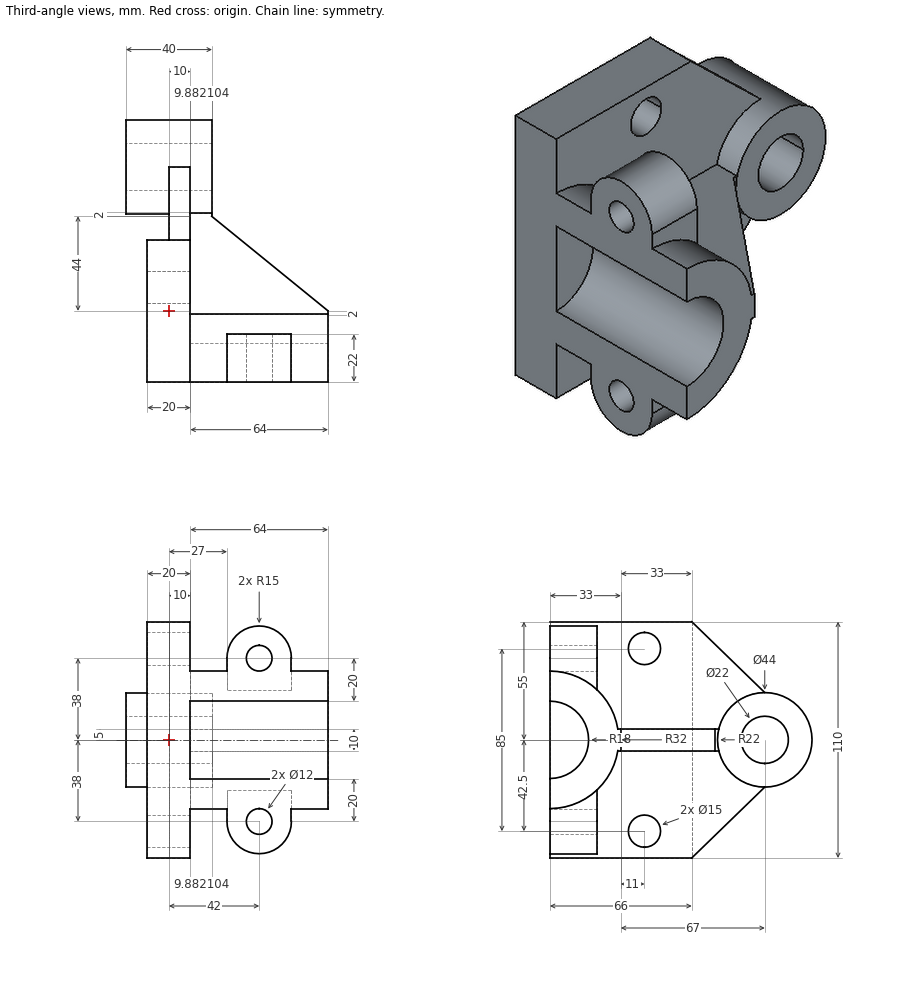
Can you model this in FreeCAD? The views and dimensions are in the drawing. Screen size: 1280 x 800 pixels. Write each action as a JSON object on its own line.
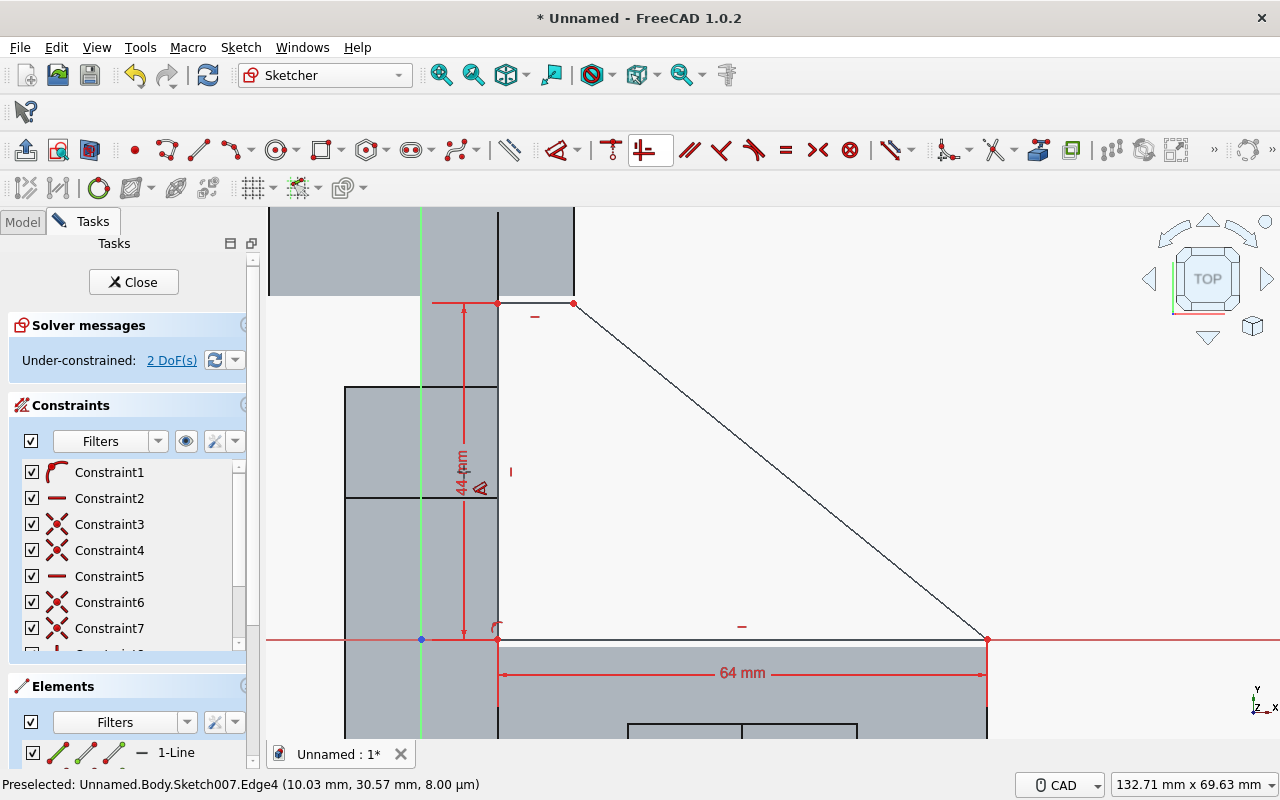
{"action": "left_click", "coordinate": [498, 640]}
{"action": "left_click", "coordinate": [460, 674]}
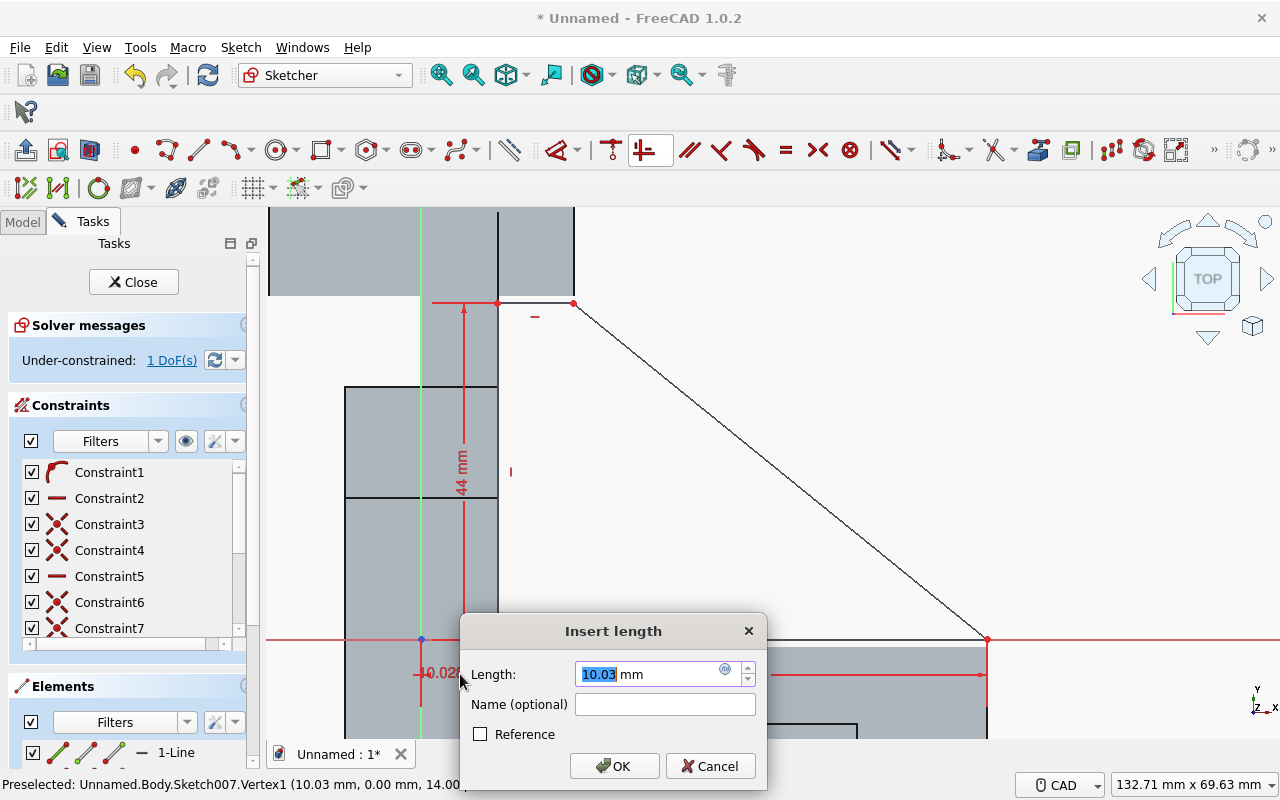
{"action": "type", "text": "10"}
{"action": "key", "text": "Return"}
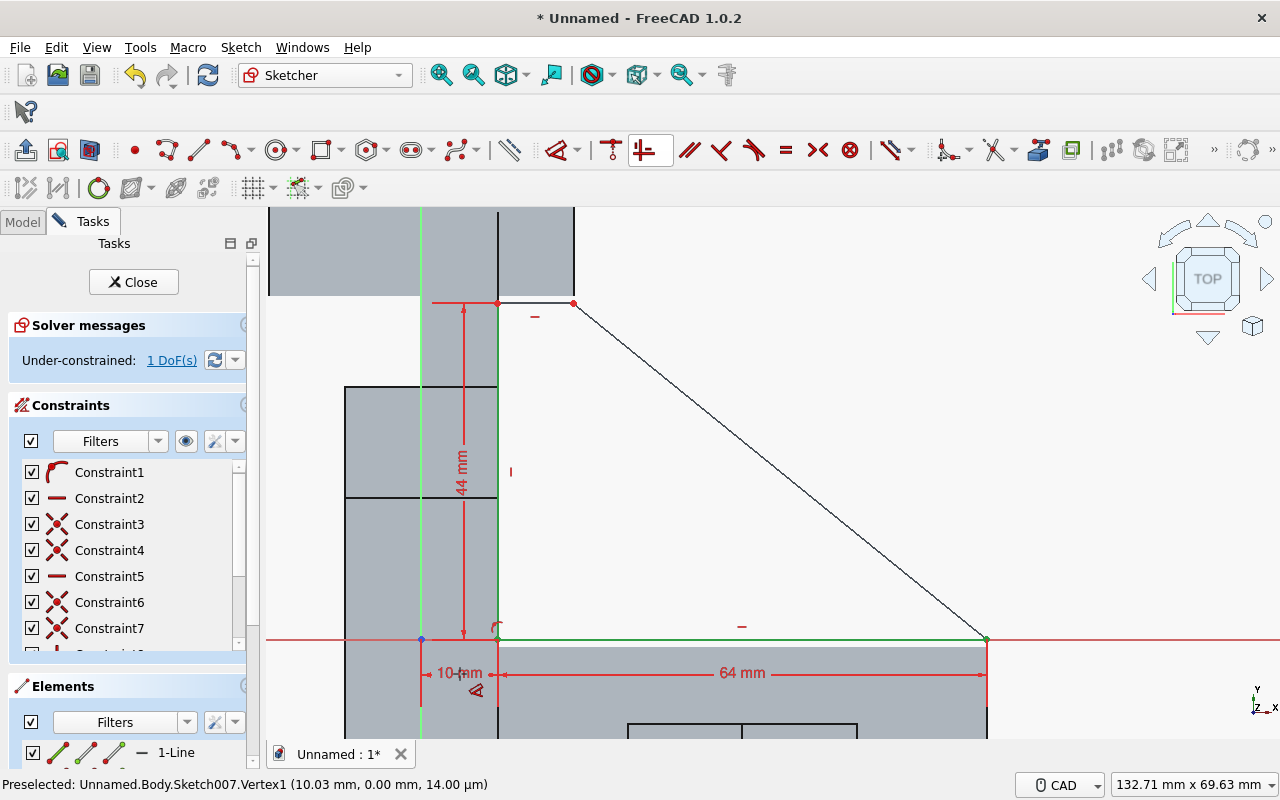
{"action": "left_click", "coordinate": [550, 303]}
{"action": "left_click", "coordinate": [535, 269]}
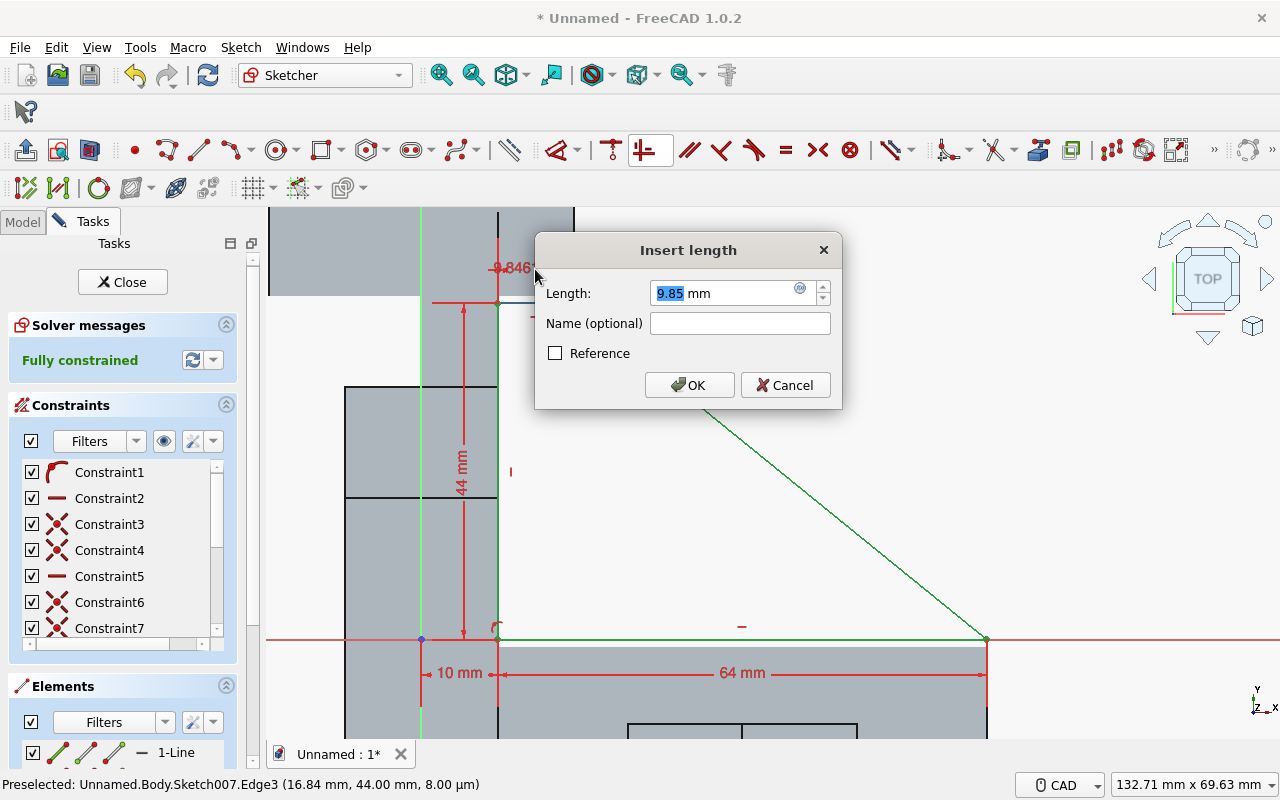
{"action": "type", "text": "9.882104"}
{"action": "key", "text": "Return"}
{"action": "key", "text": "Escape"}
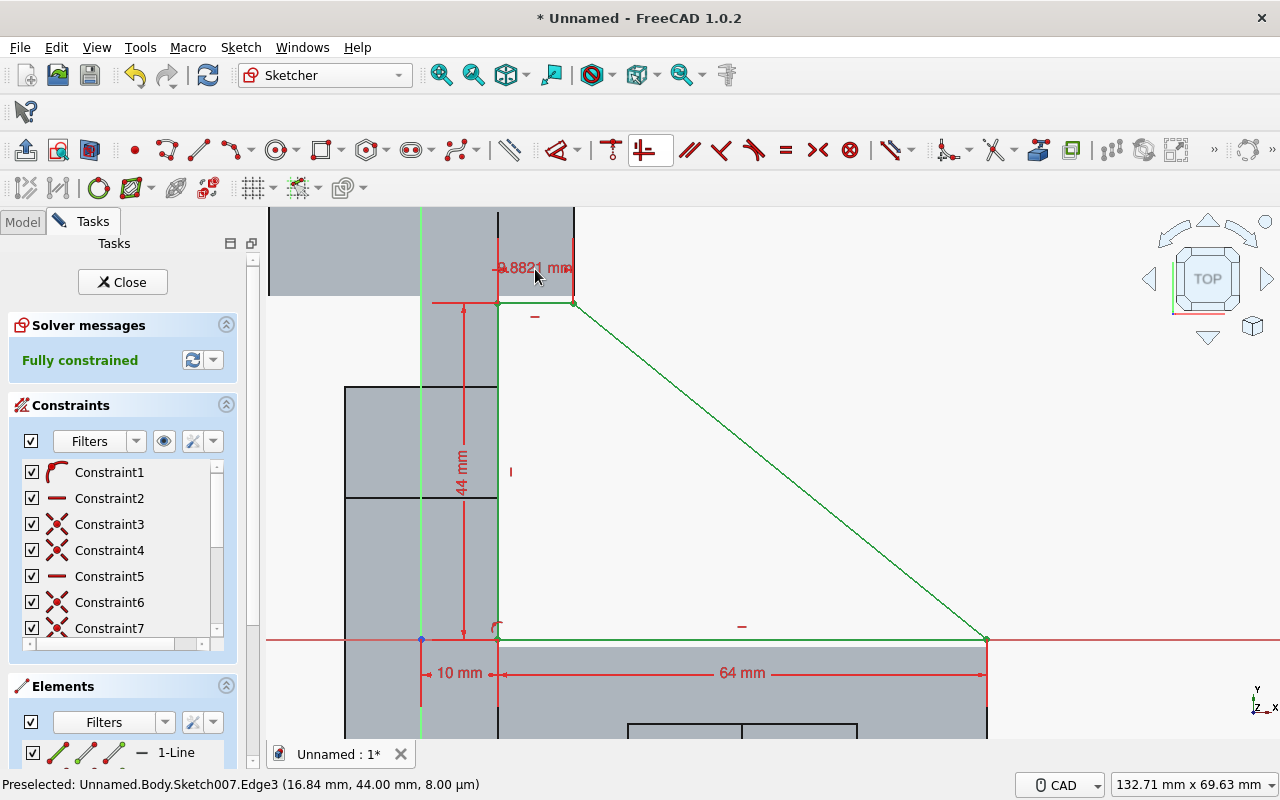
{"action": "left_click", "coordinate": [123, 282]}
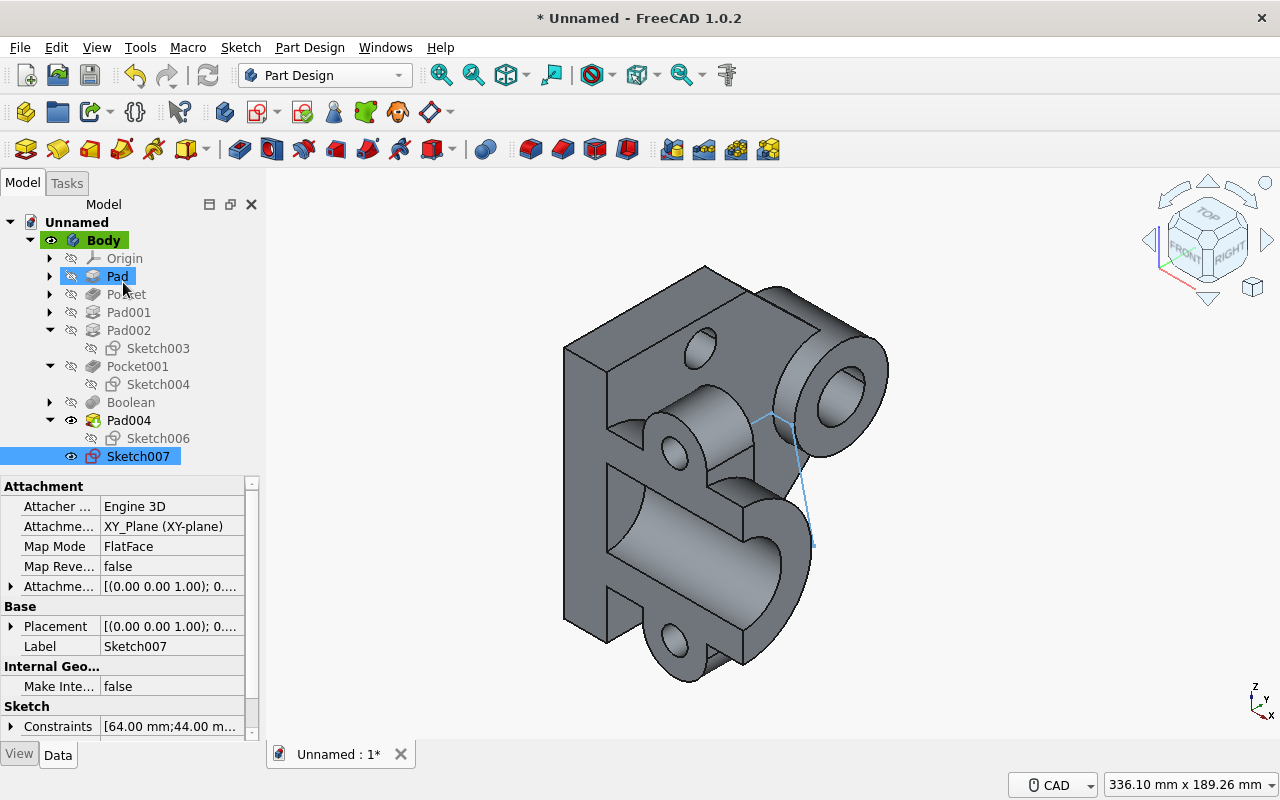
{"action": "left_click", "coordinate": [26, 150]}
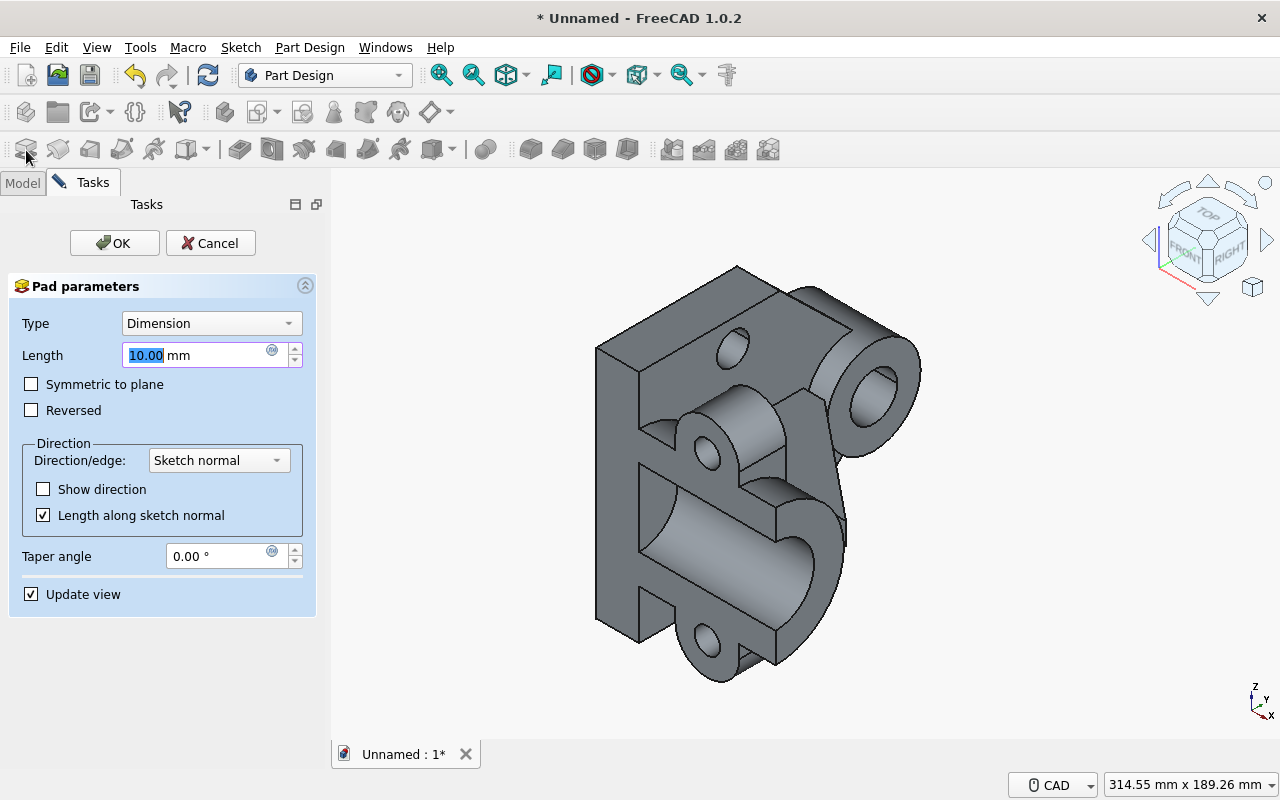
{"action": "type", "text": "10"}
{"action": "key", "text": "Tab"}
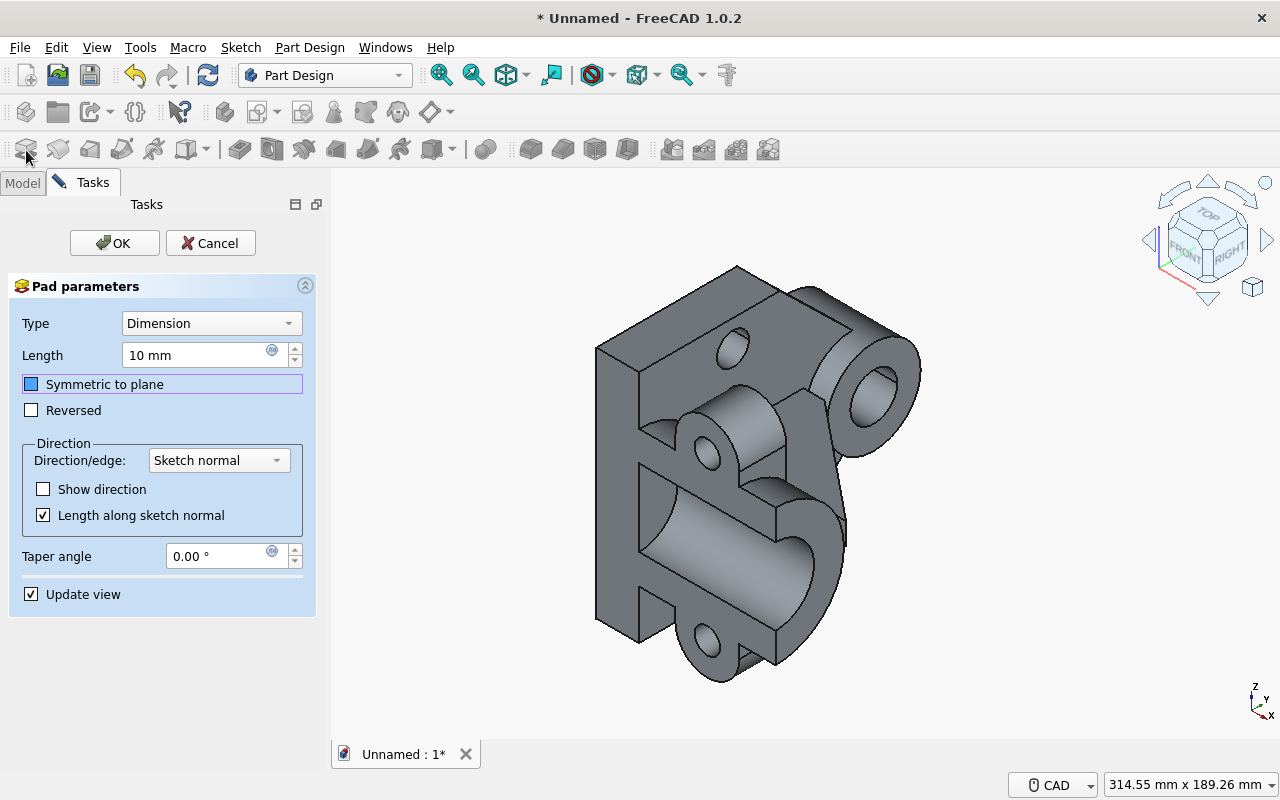
{"action": "left_click", "coordinate": [30, 384]}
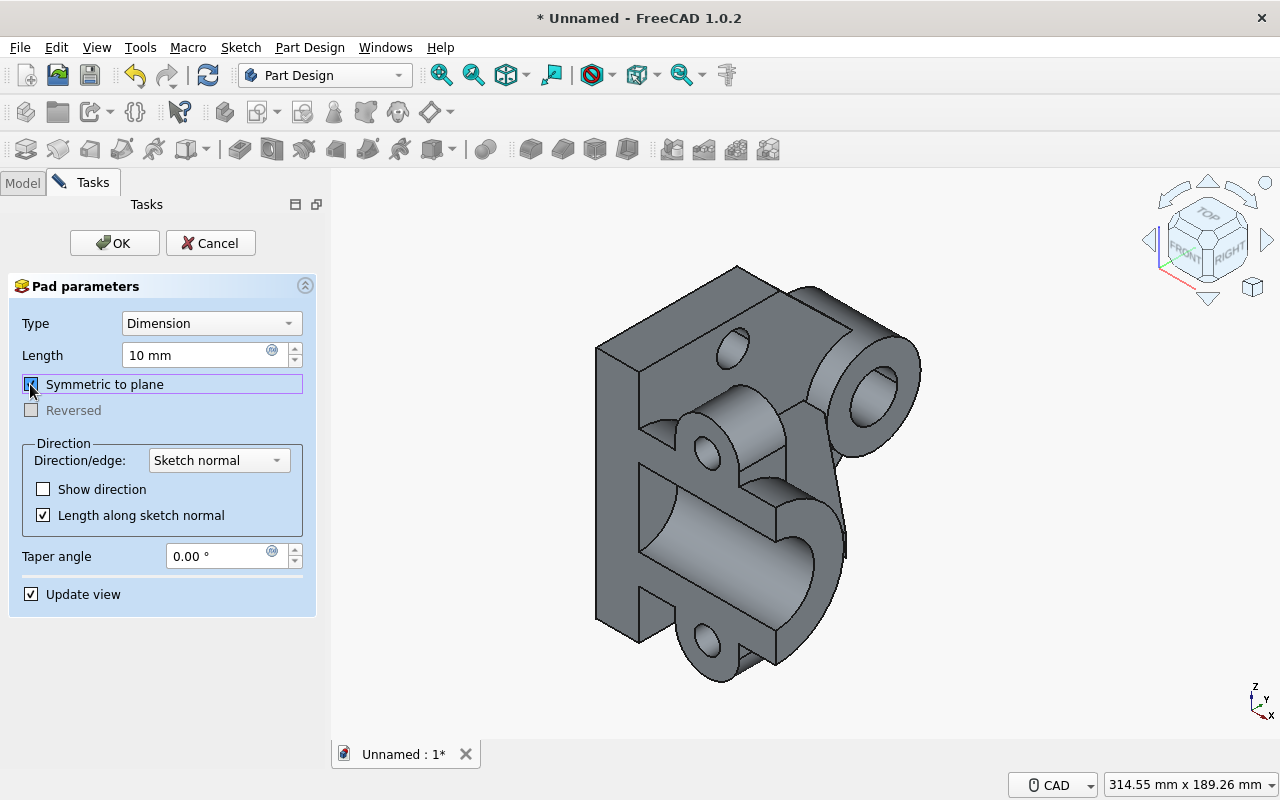
{"action": "left_click", "coordinate": [115, 243]}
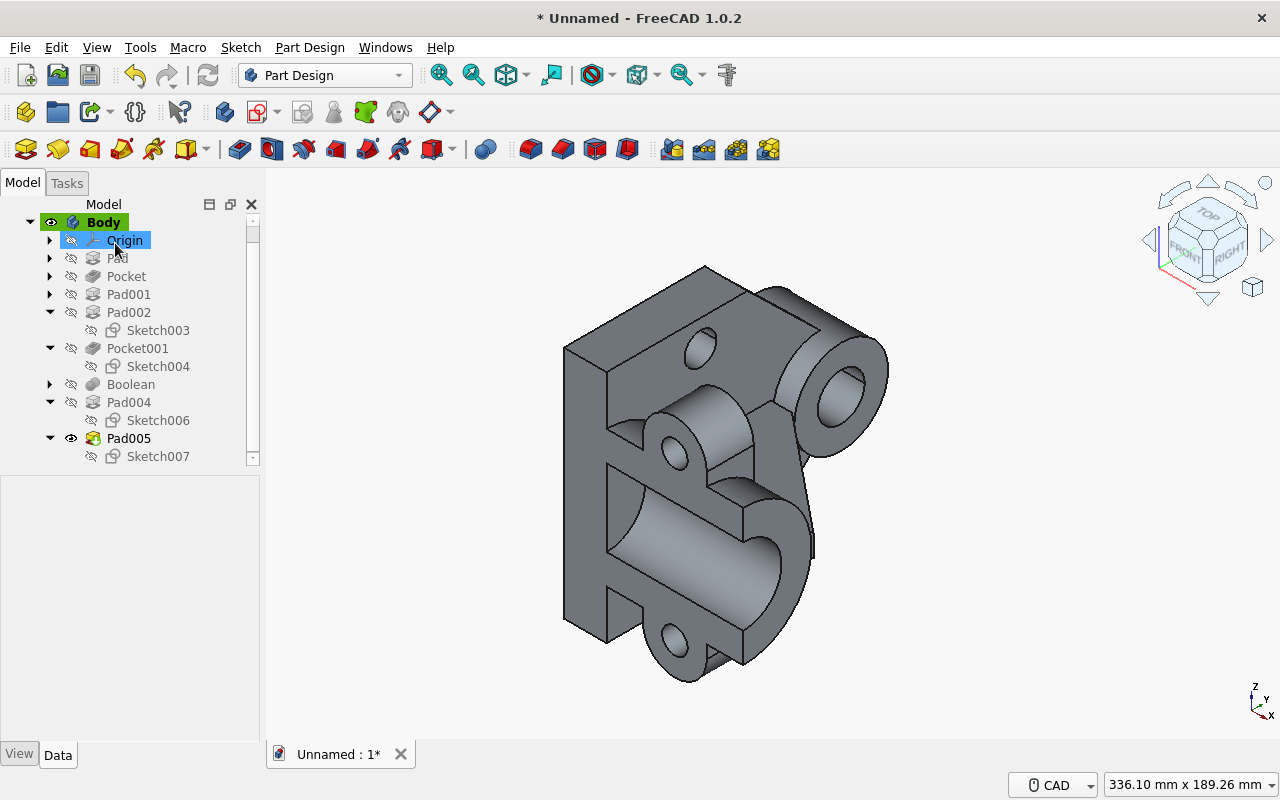
{"action": "left_click", "coordinate": [50, 240]}